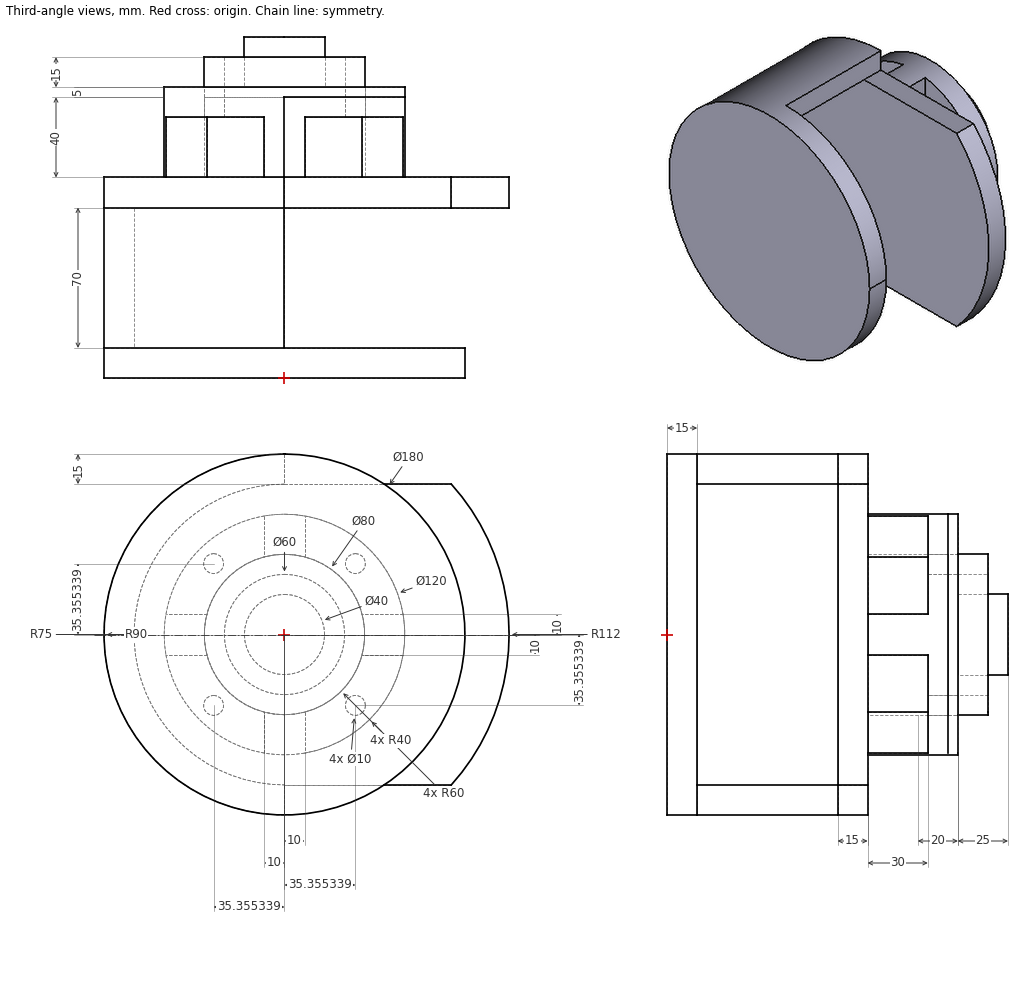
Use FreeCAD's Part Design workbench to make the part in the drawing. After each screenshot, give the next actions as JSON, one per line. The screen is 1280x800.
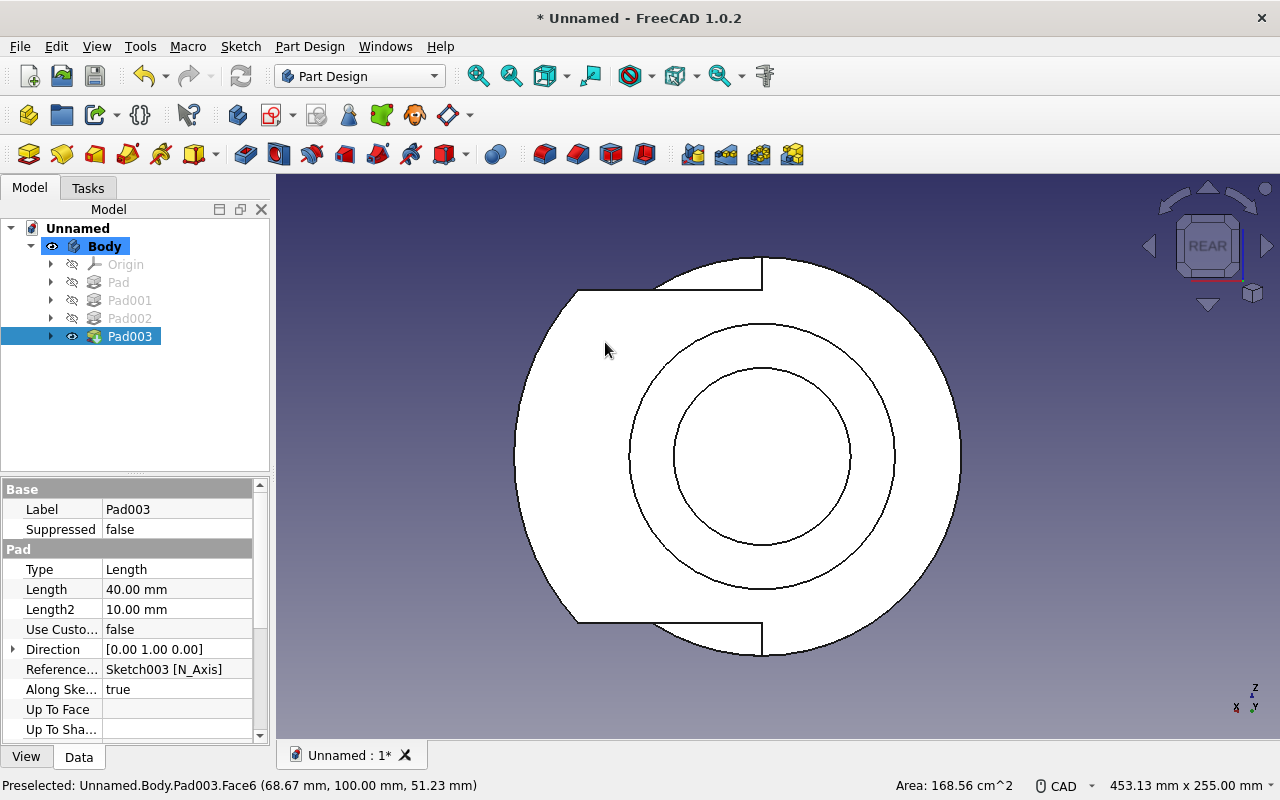
{"action": "left_click", "coordinate": [270, 116]}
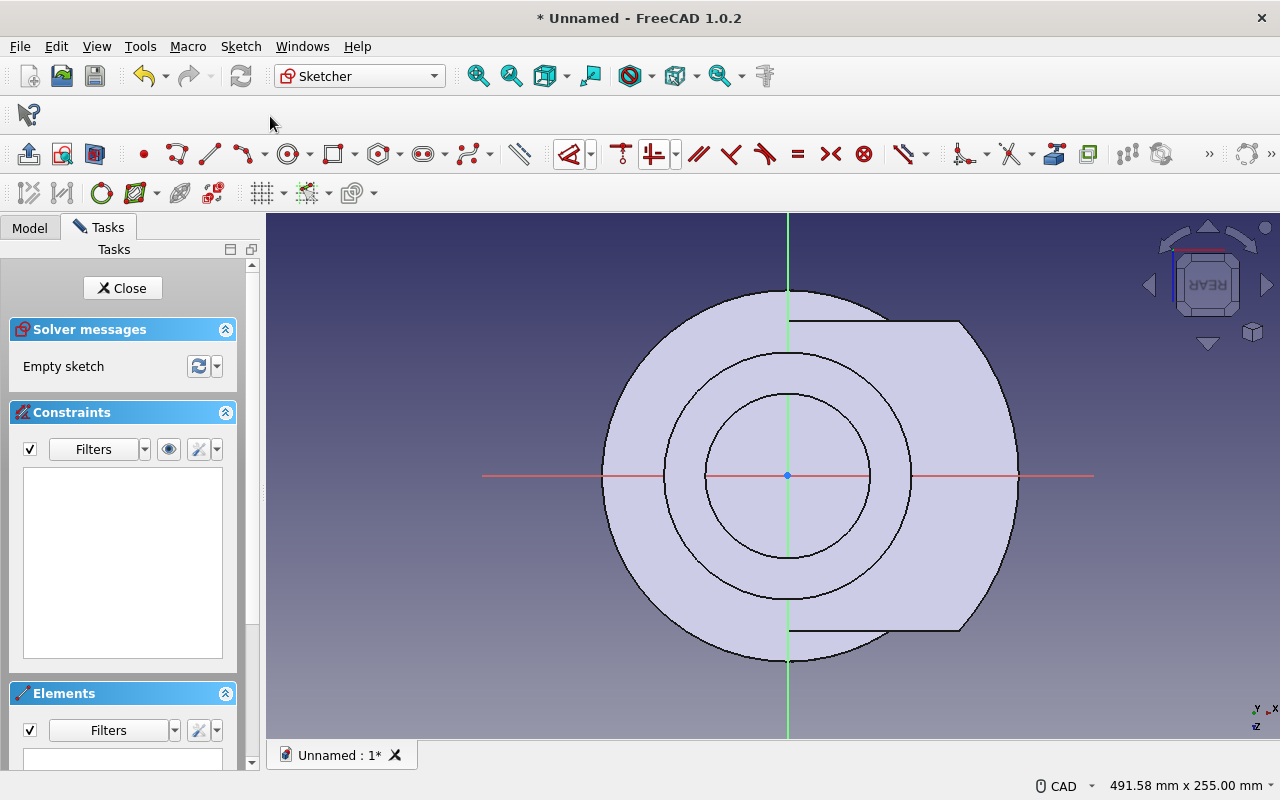
{"action": "scroll", "coordinate": [957, 476], "scroll_direction": "up", "scroll_amount": 2}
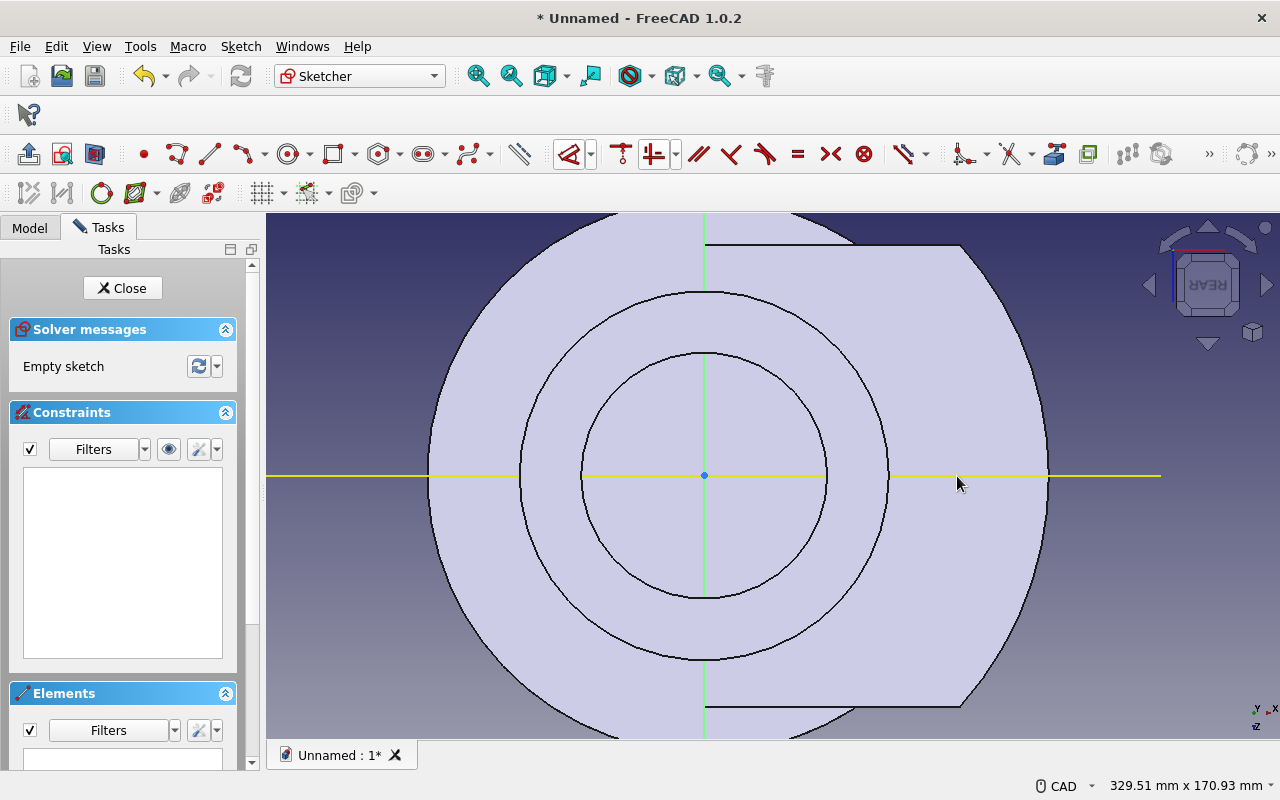
{"action": "key", "text": "g l"}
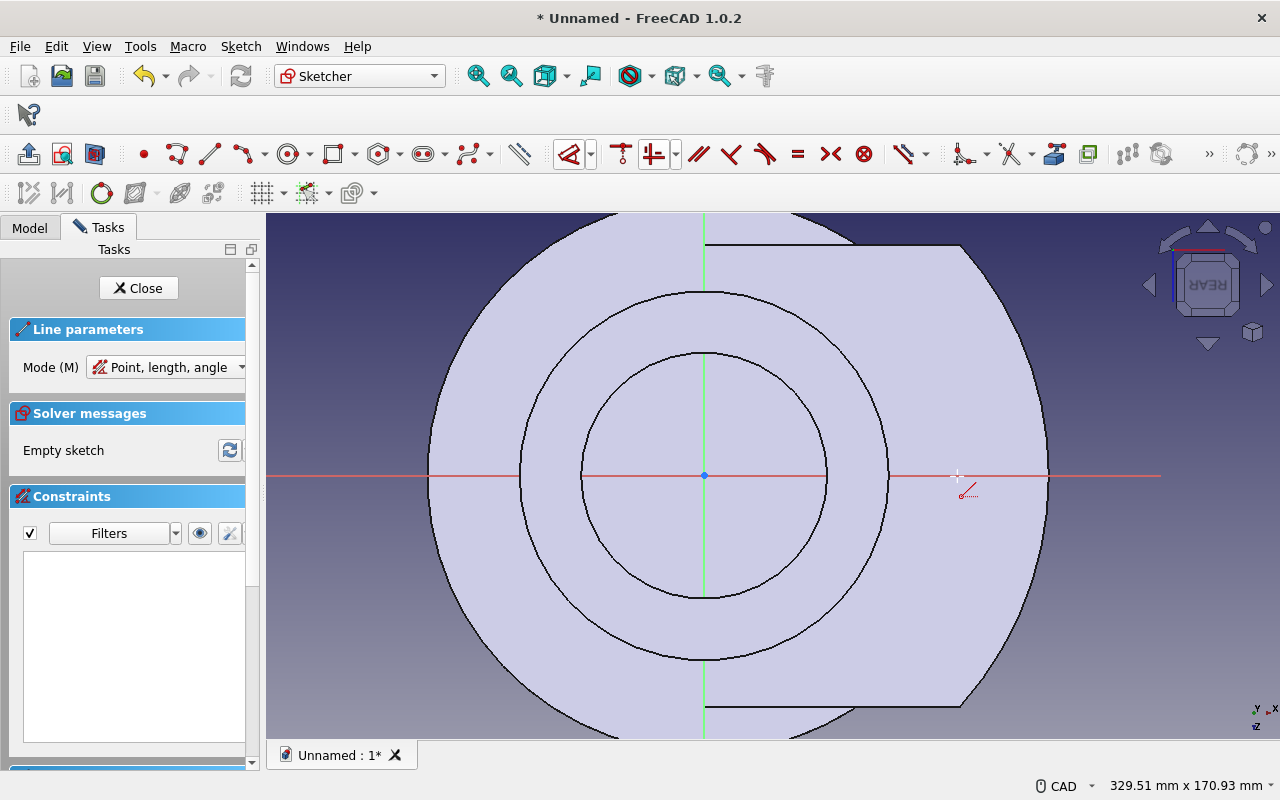
{"action": "left_click", "coordinate": [823, 445]}
{"action": "left_click", "coordinate": [886, 445]}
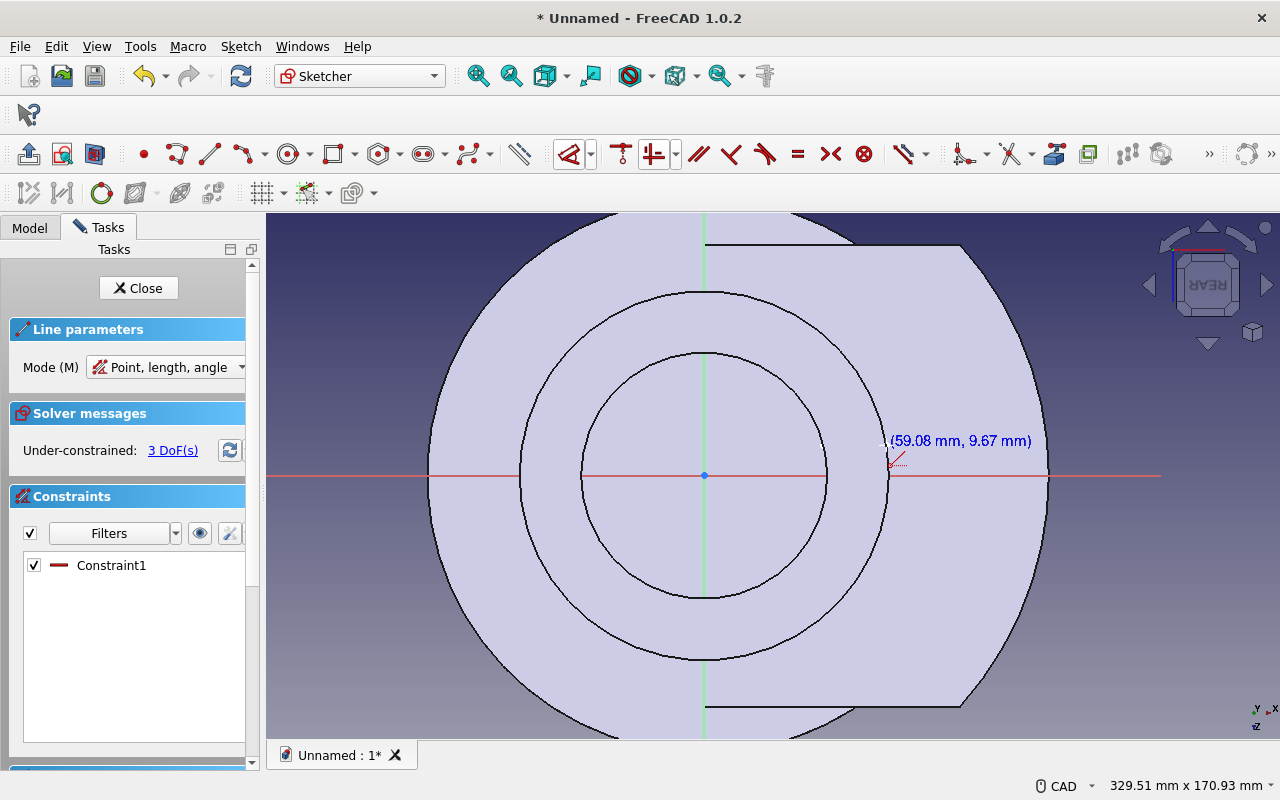
{"action": "left_click", "coordinate": [735, 294]}
{"action": "left_click", "coordinate": [735, 357]}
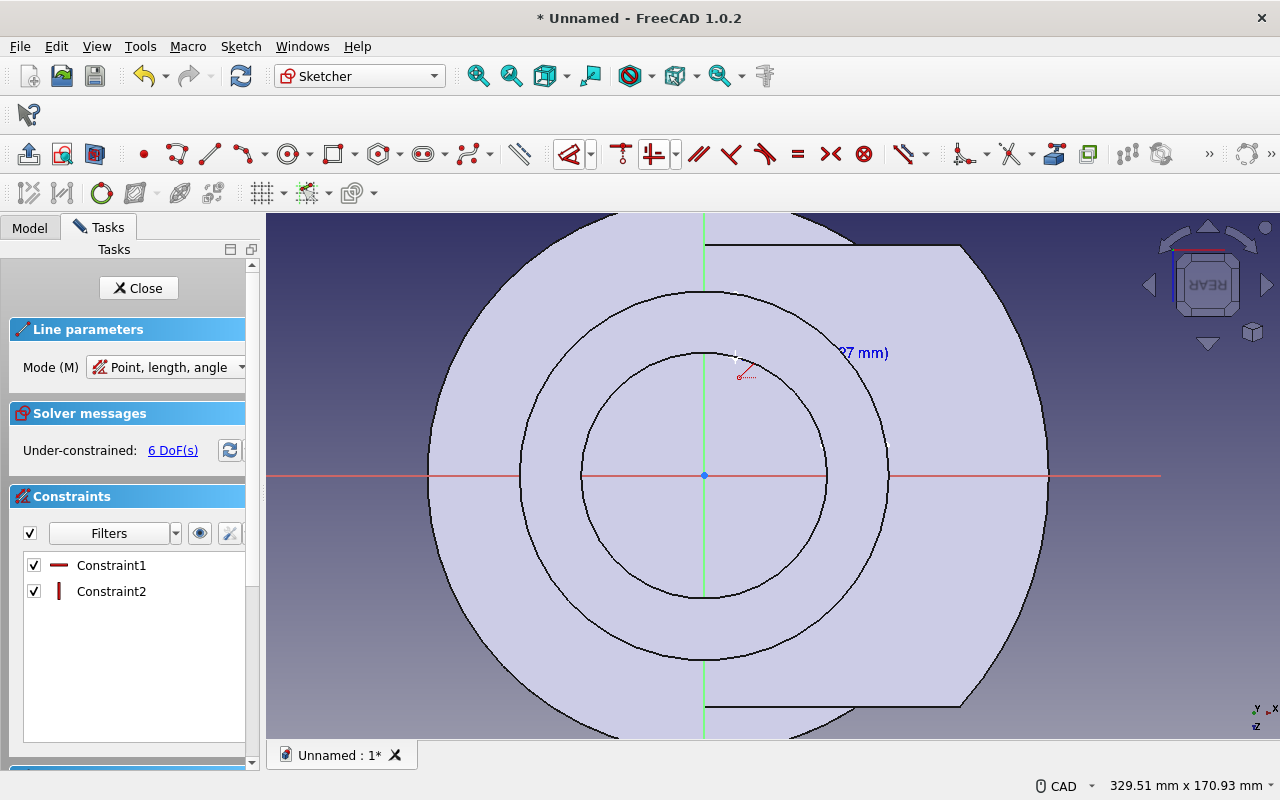
{"action": "key", "text": "g 3 a"}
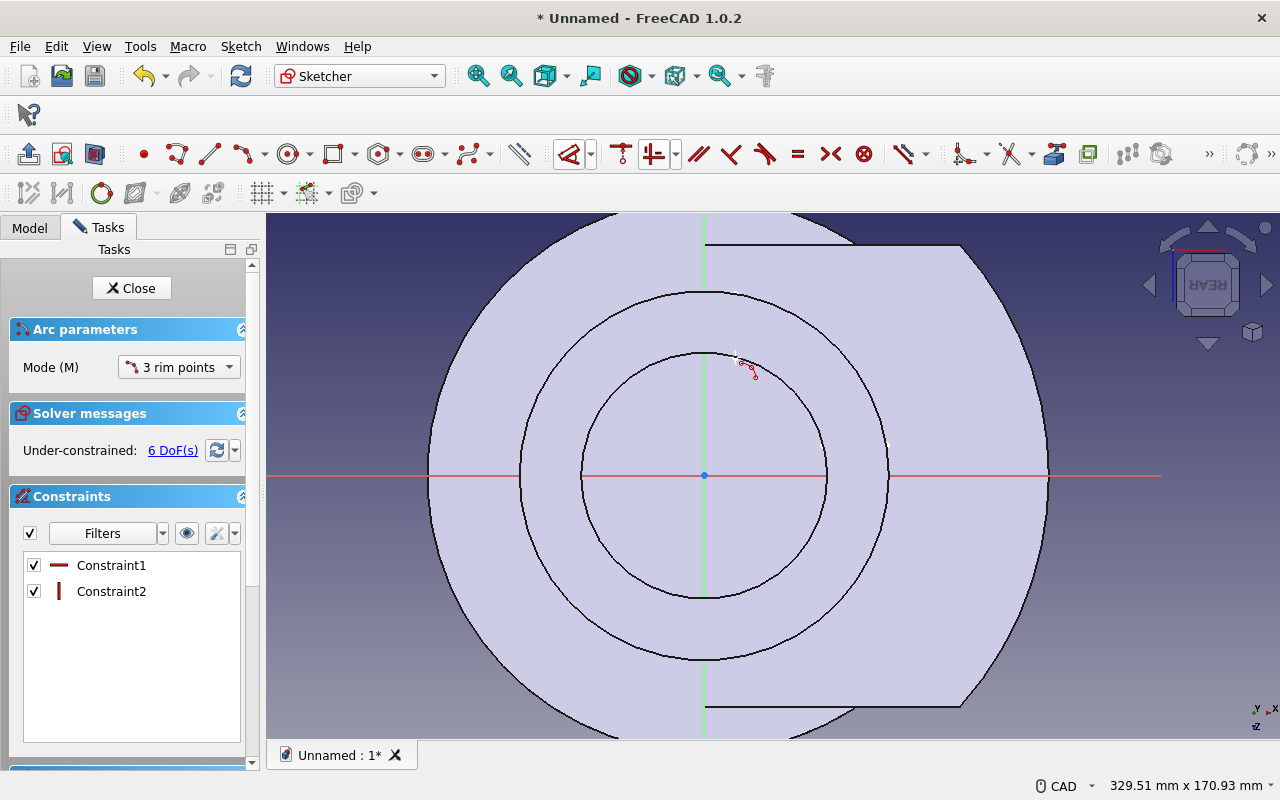
{"action": "left_click", "coordinate": [886, 446]}
{"action": "left_click", "coordinate": [735, 295]}
{"action": "left_click", "coordinate": [835, 345]}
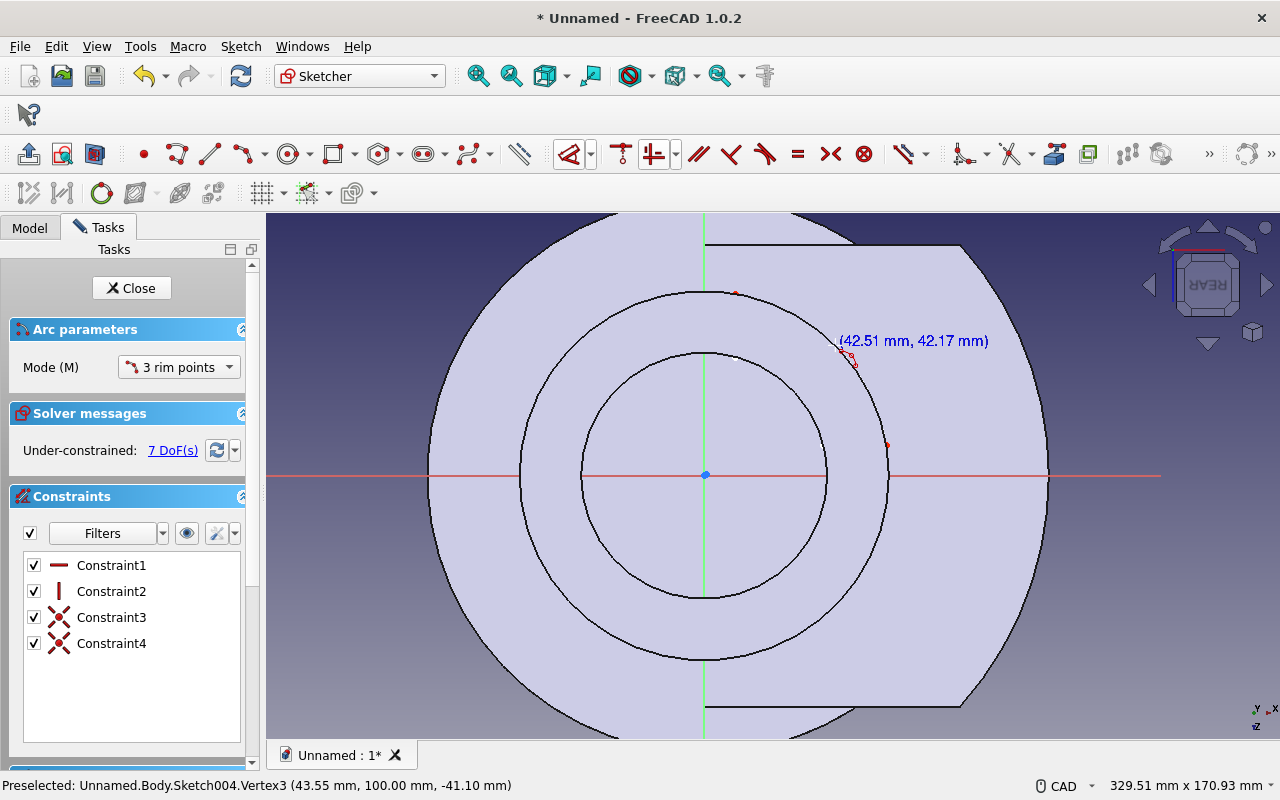
{"action": "left_click", "coordinate": [735, 358]}
{"action": "left_click", "coordinate": [823, 446]}
{"action": "left_click", "coordinate": [791, 389]}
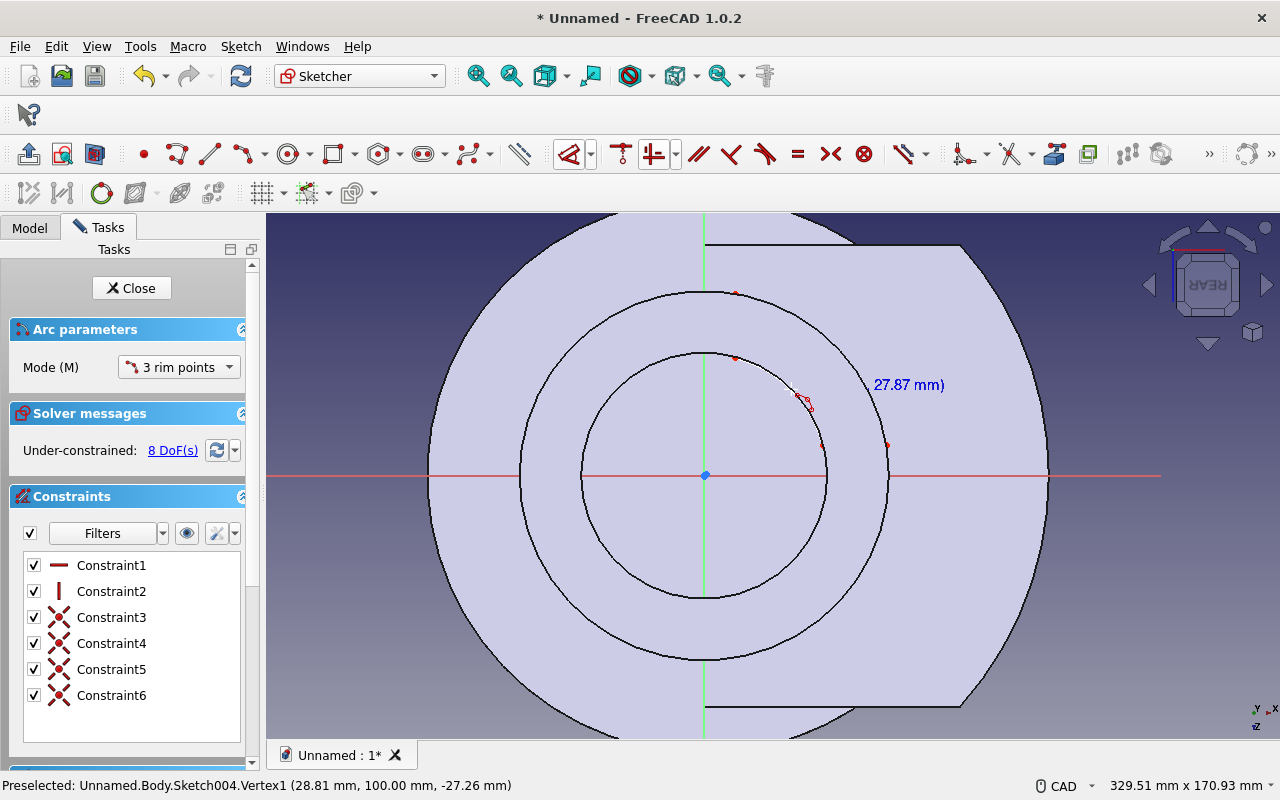
{"action": "left_click", "coordinate": [210, 154]}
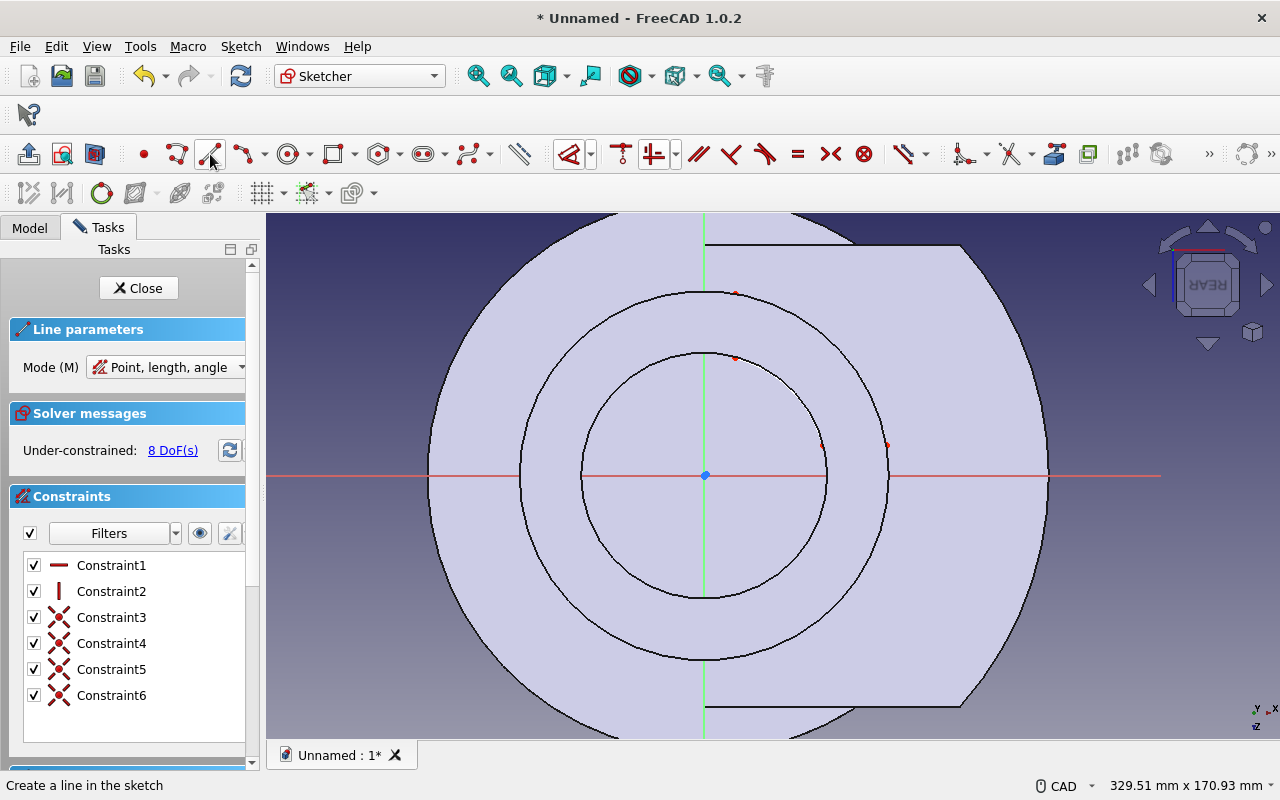
{"action": "left_click", "coordinate": [673, 357]}
{"action": "left_click", "coordinate": [673, 294]}